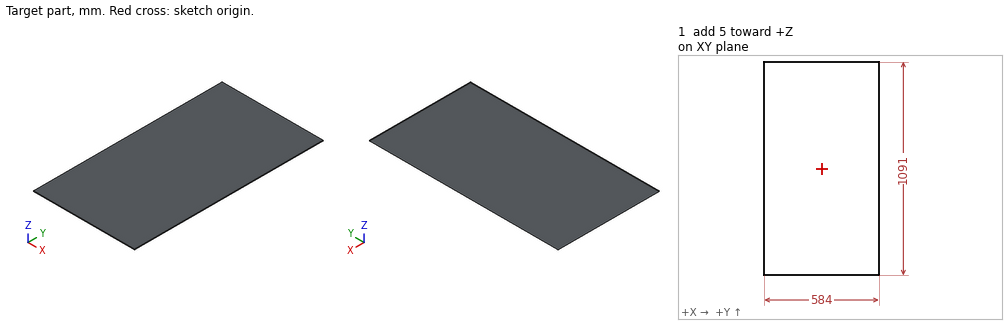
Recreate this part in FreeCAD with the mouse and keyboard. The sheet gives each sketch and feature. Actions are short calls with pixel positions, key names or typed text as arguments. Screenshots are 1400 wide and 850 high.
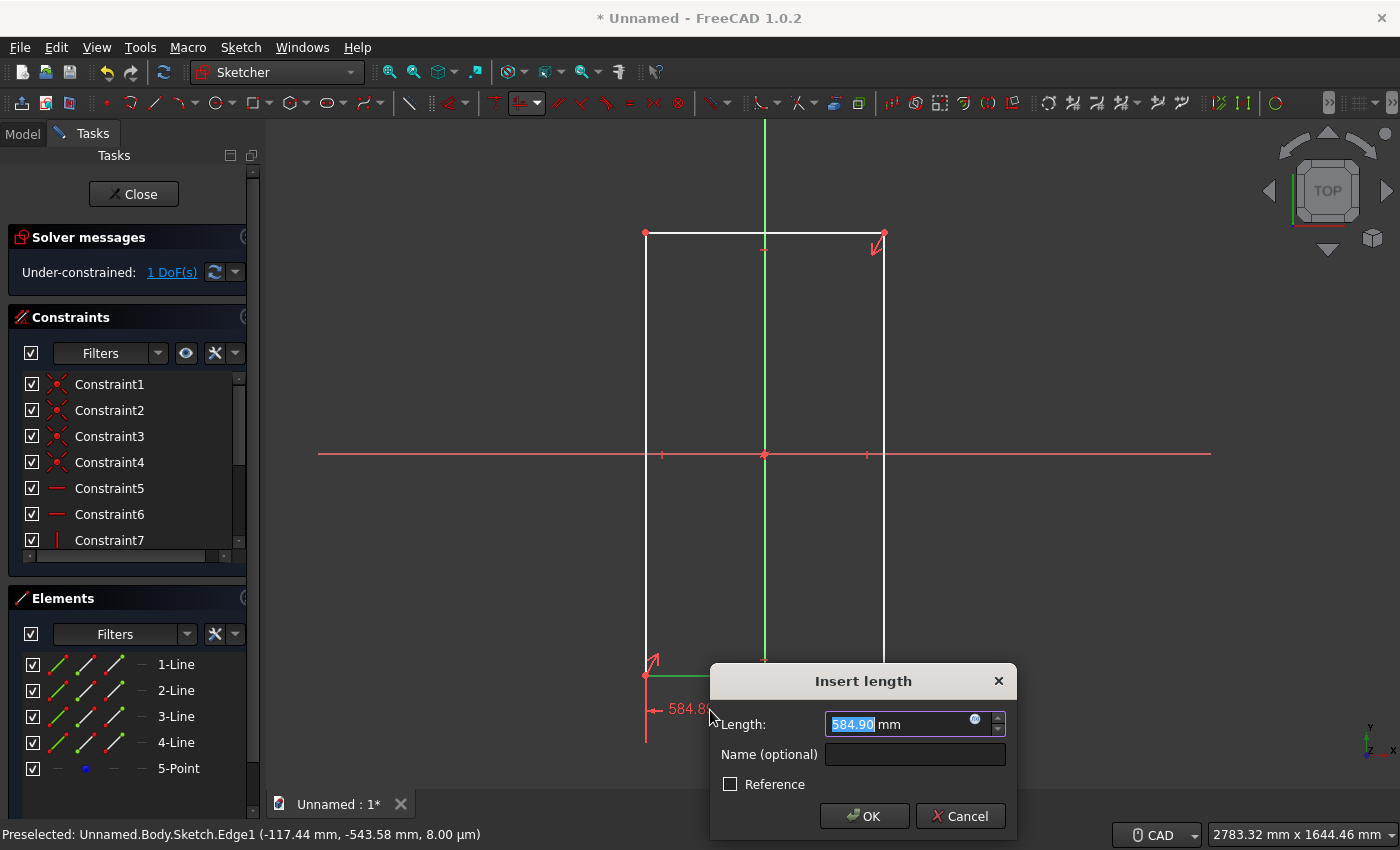
text(584)
key(Return)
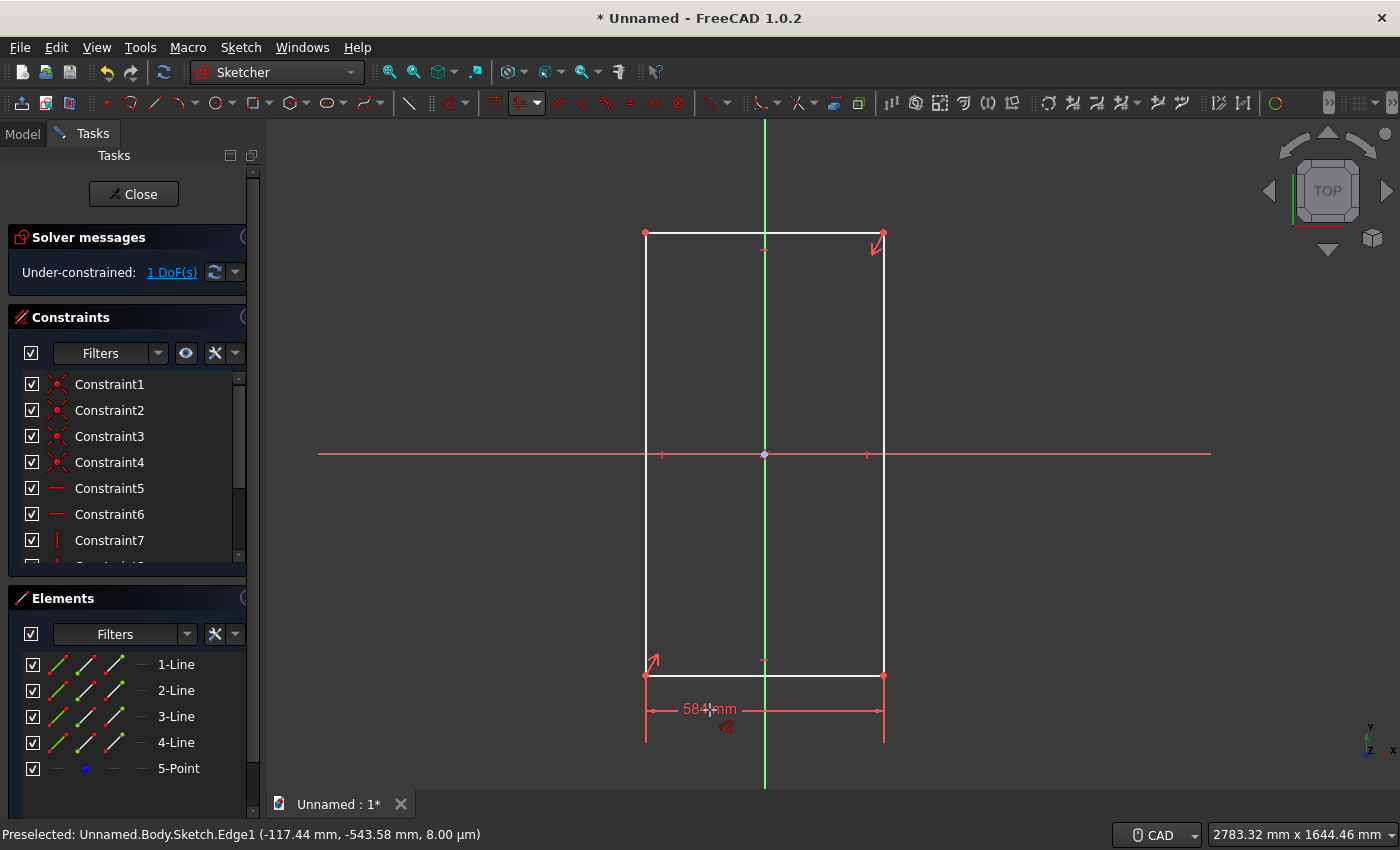
click(884, 543)
click(918, 353)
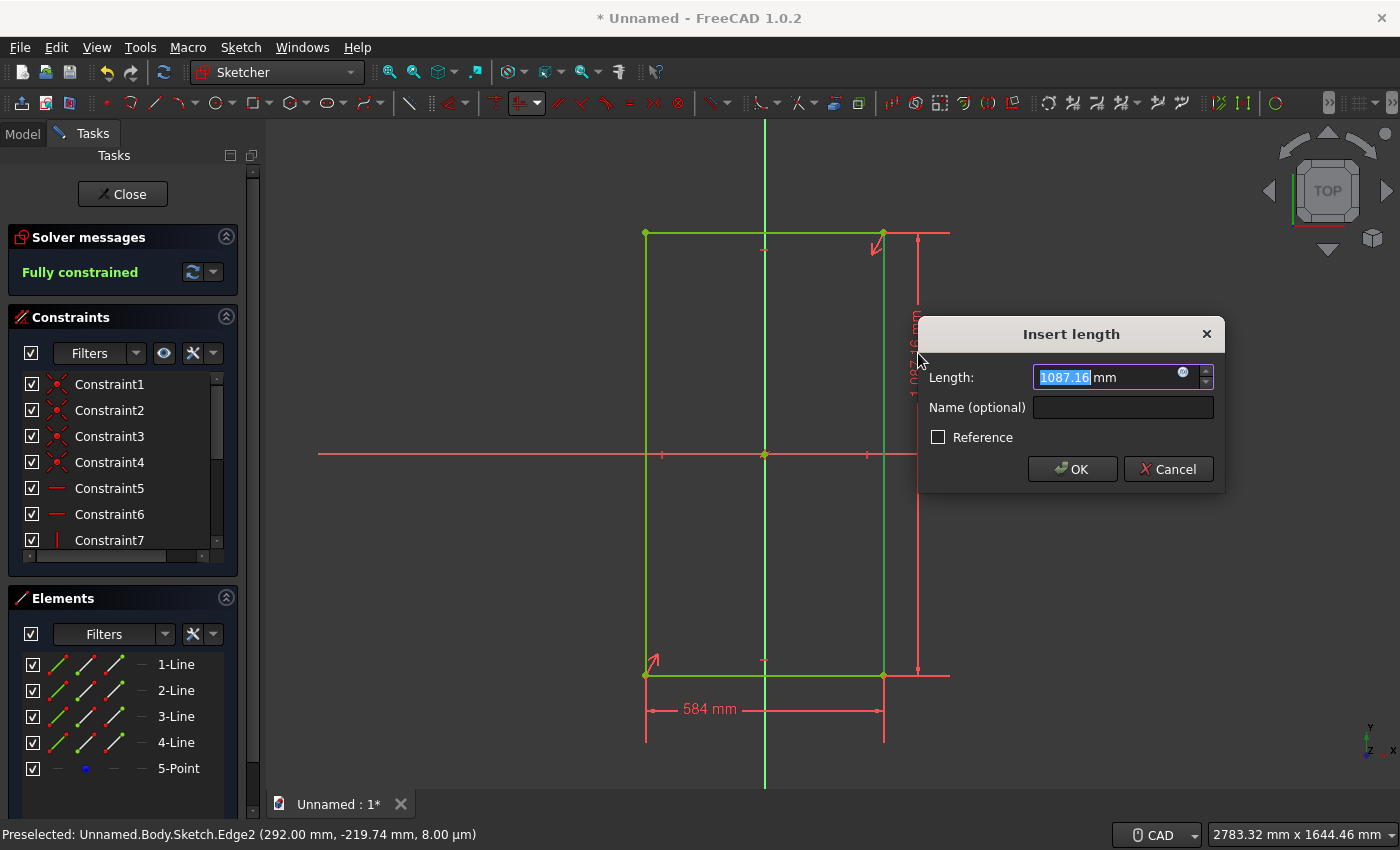
text(1091)
key(Return)
key(Escape)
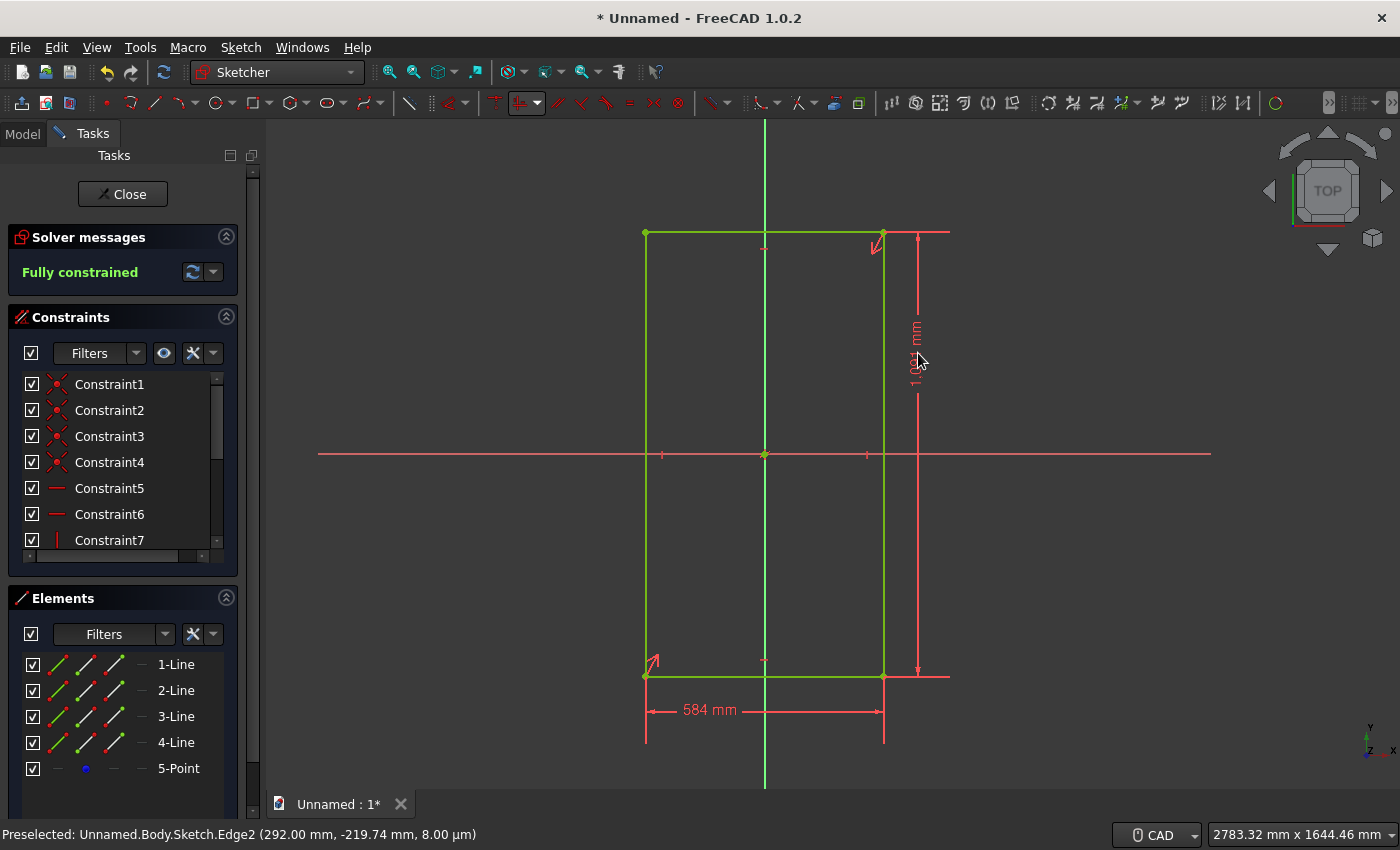
click(123, 194)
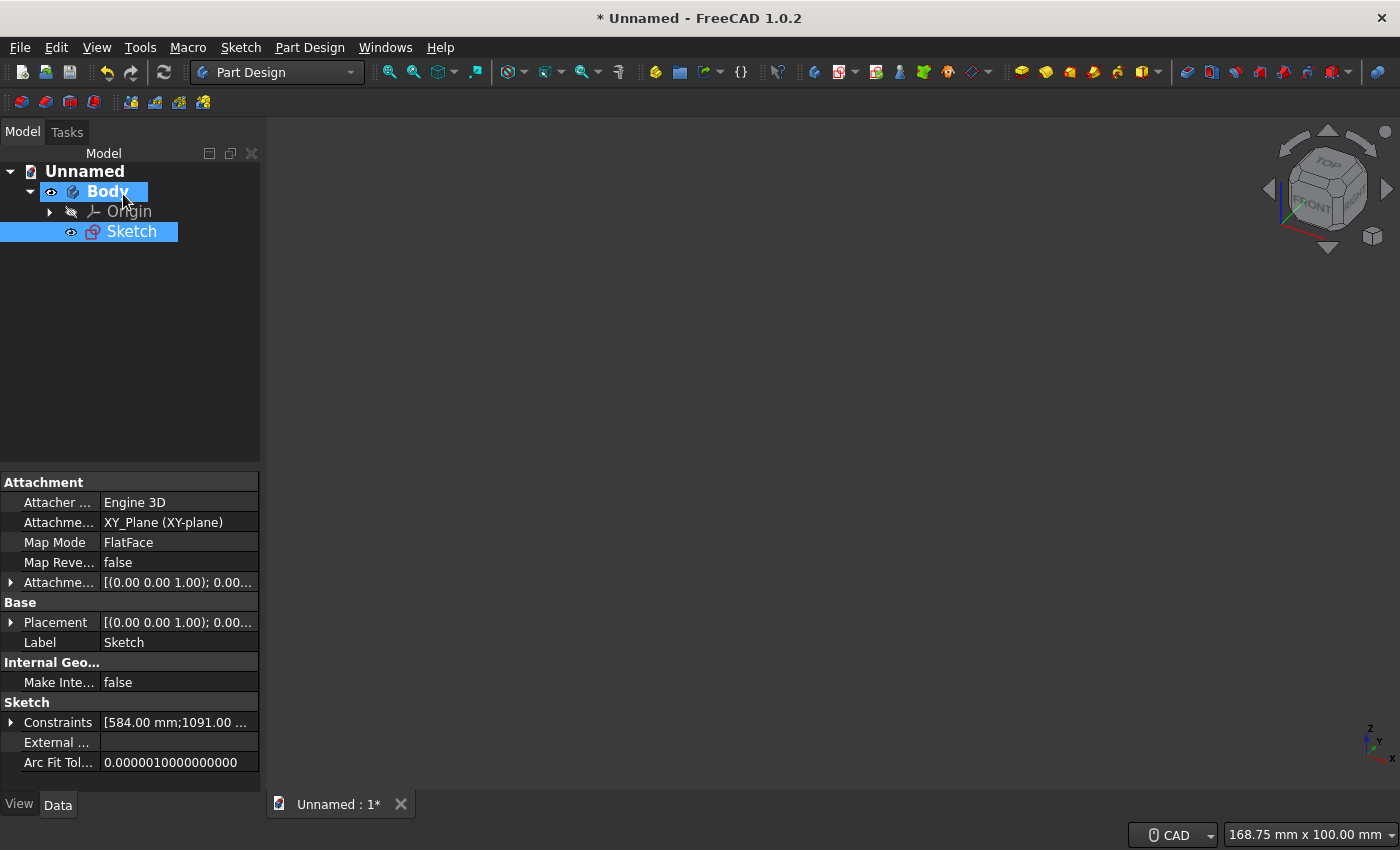
click(1022, 72)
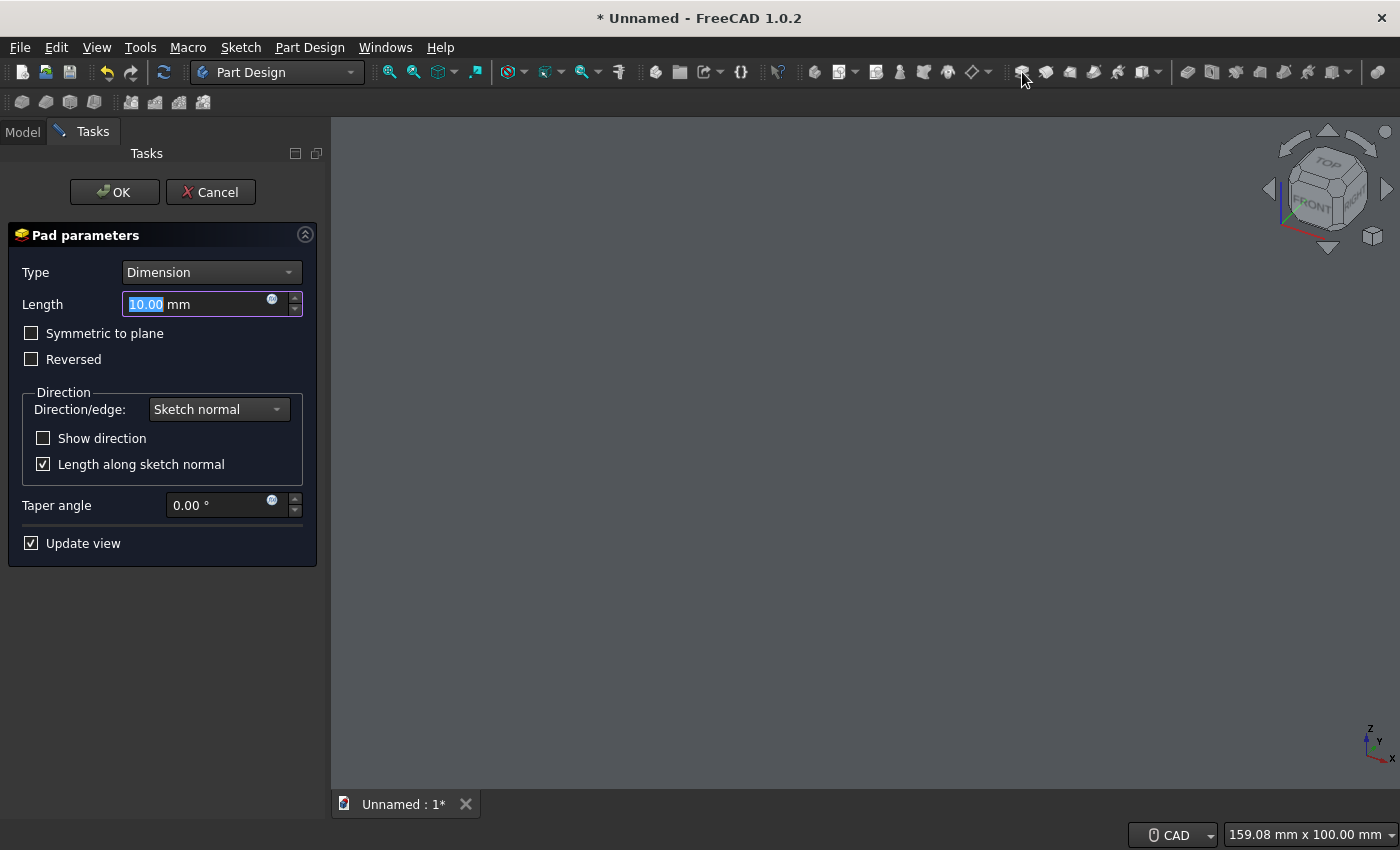
text(5)
key(Tab)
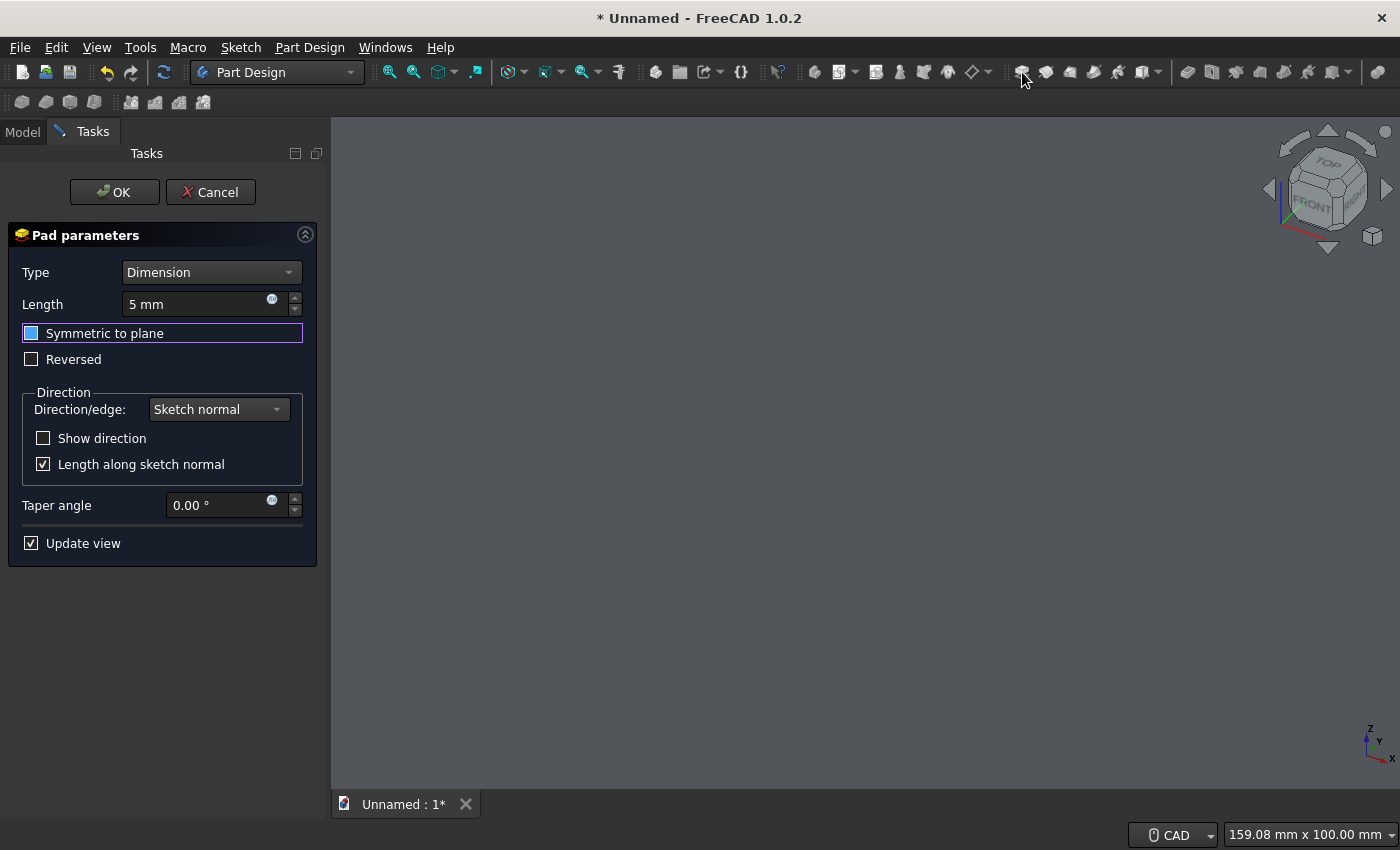
click(115, 192)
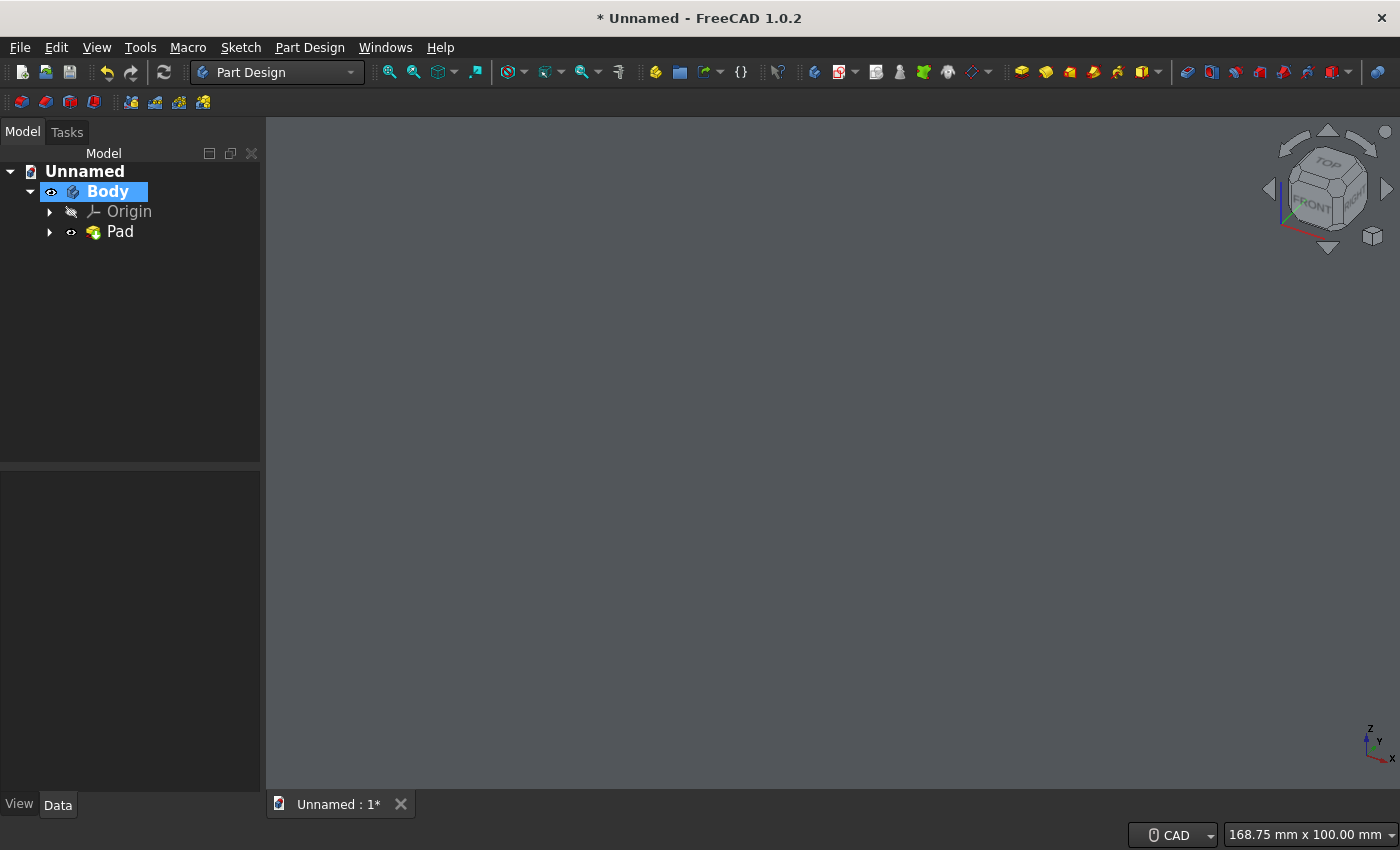
key(0)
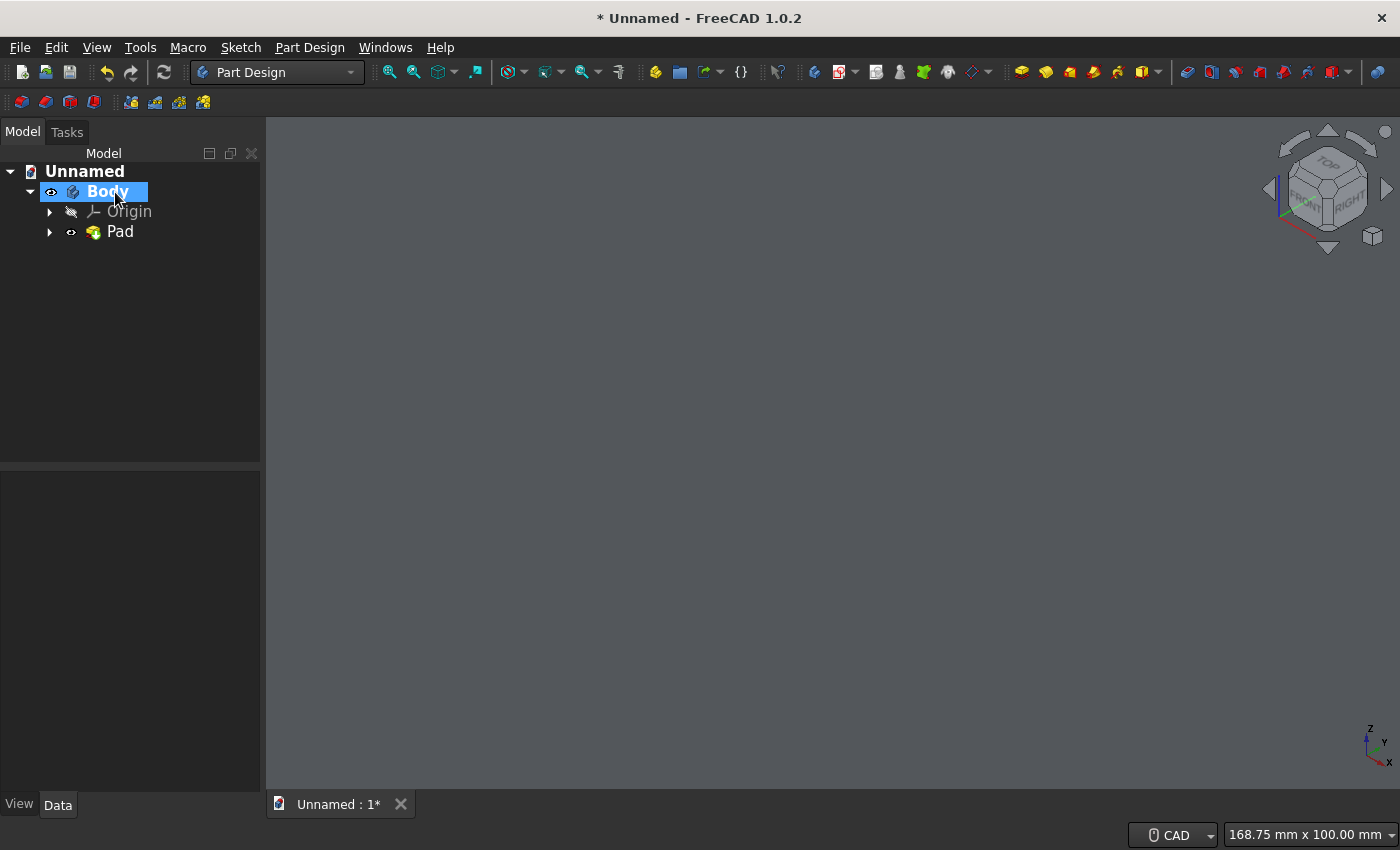
click(390, 72)